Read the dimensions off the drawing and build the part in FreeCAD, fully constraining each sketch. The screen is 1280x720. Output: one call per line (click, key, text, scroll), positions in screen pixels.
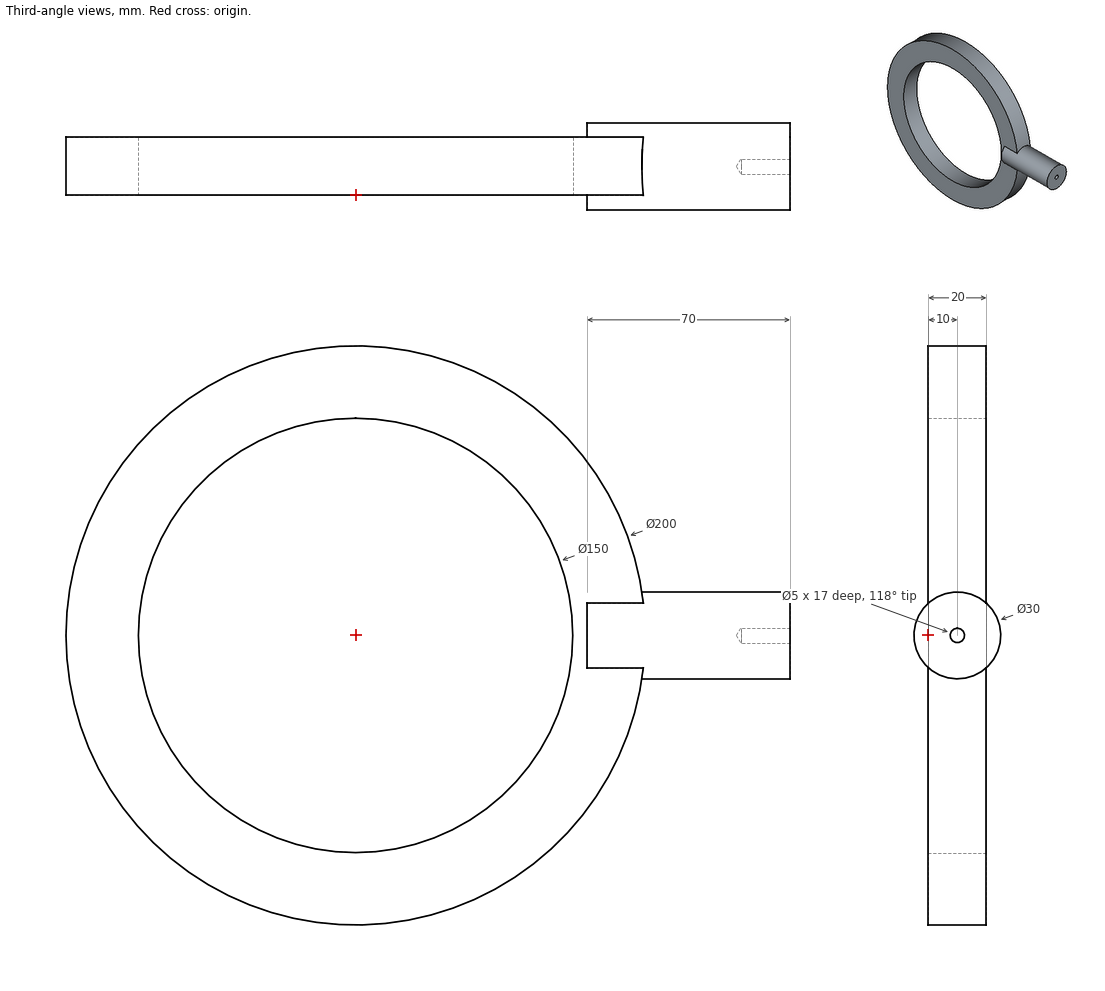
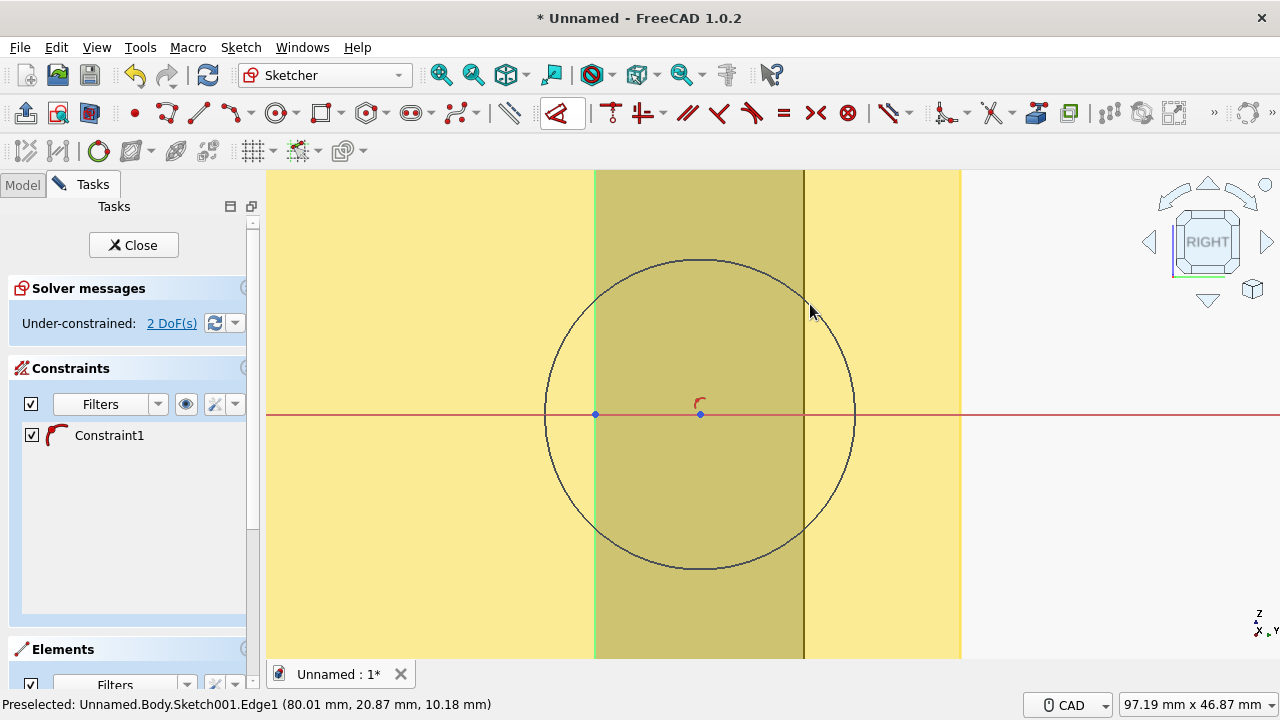
key(d)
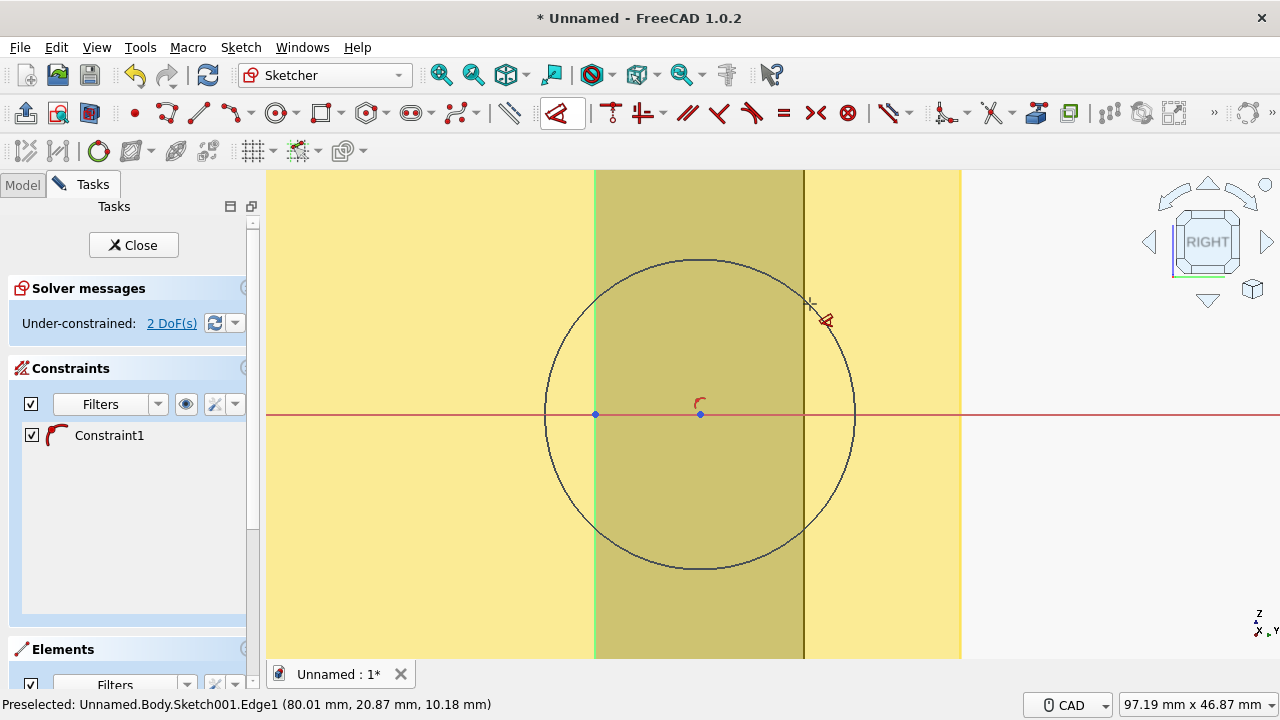
click(809, 304)
click(831, 281)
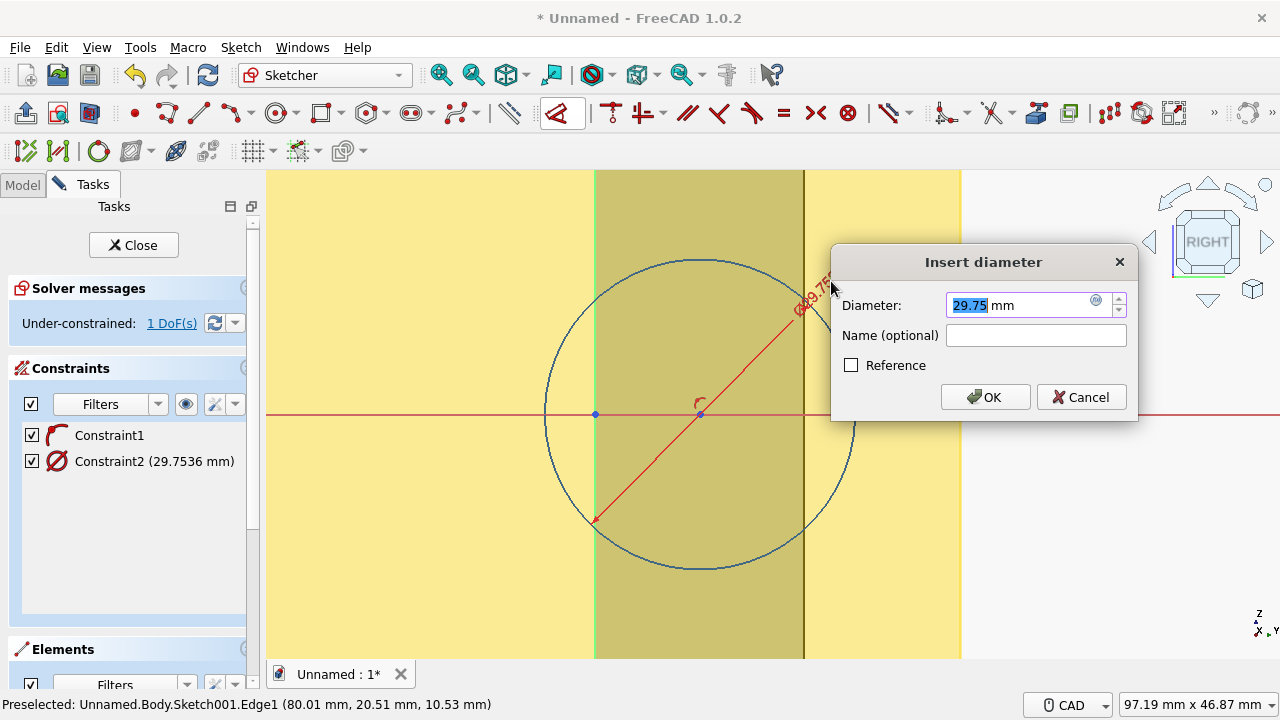
text(30)
key(Return)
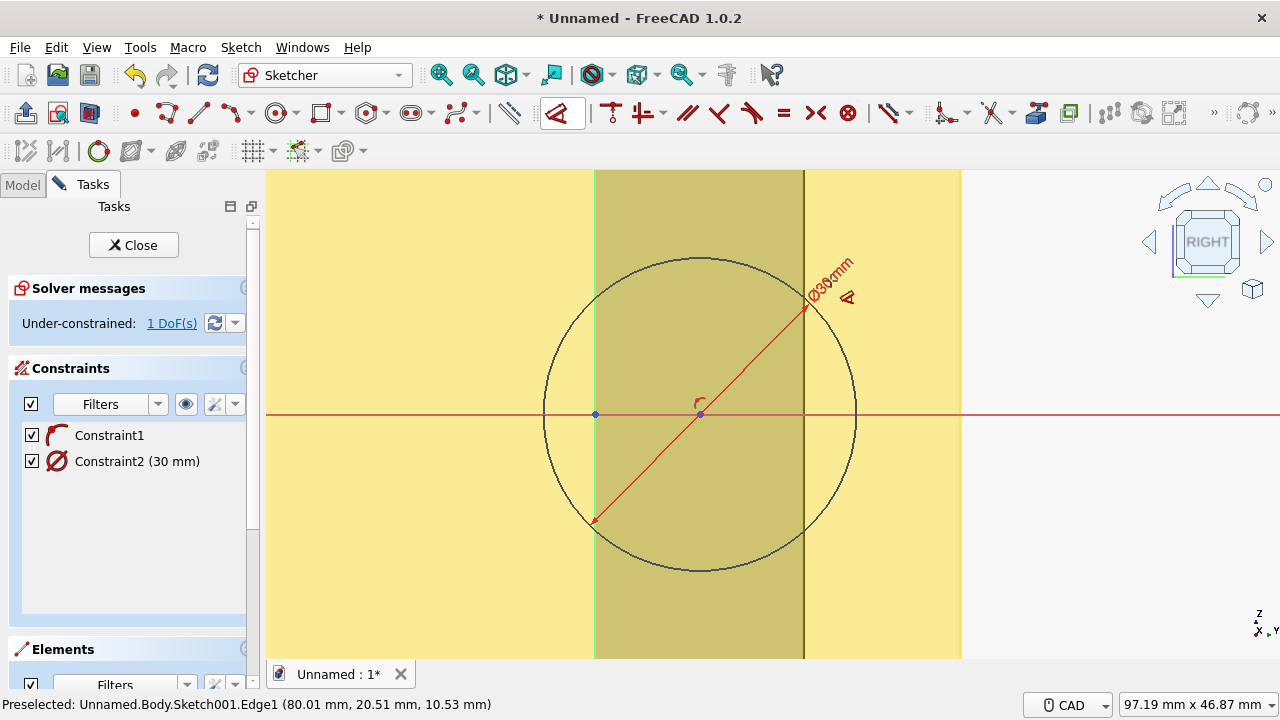
click(700, 414)
click(648, 448)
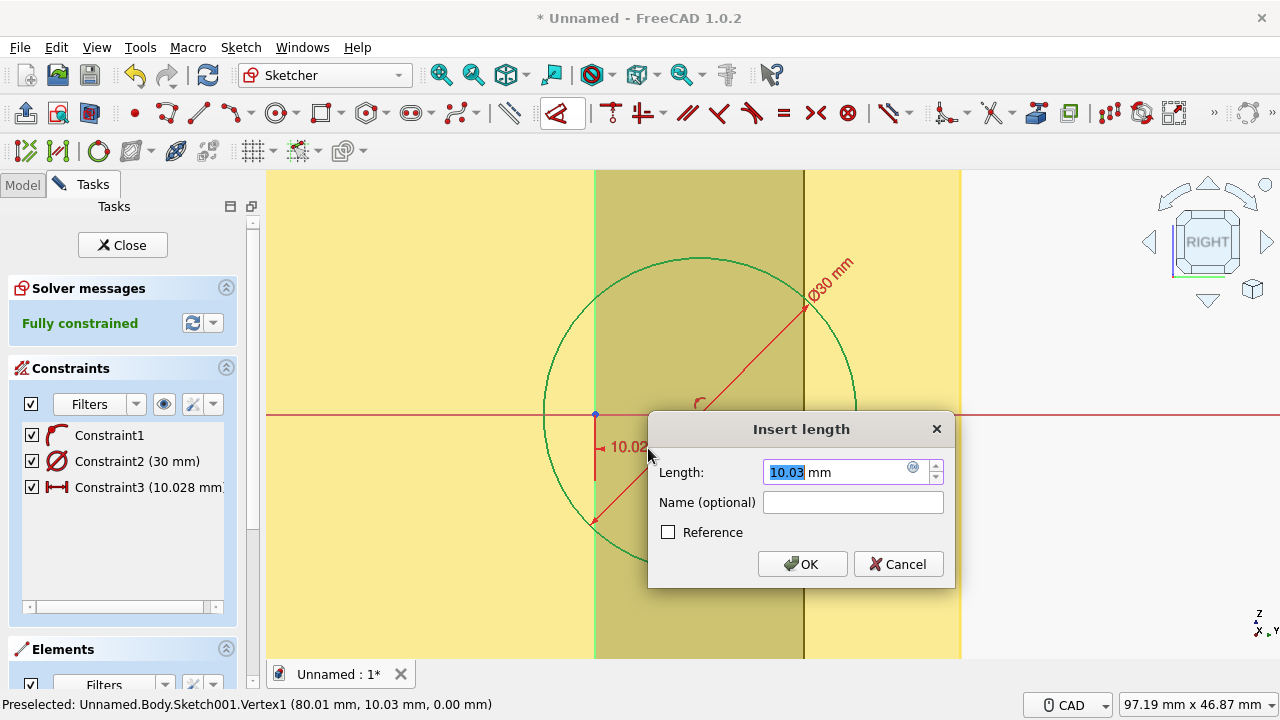
text(10)
key(Return)
key(Escape)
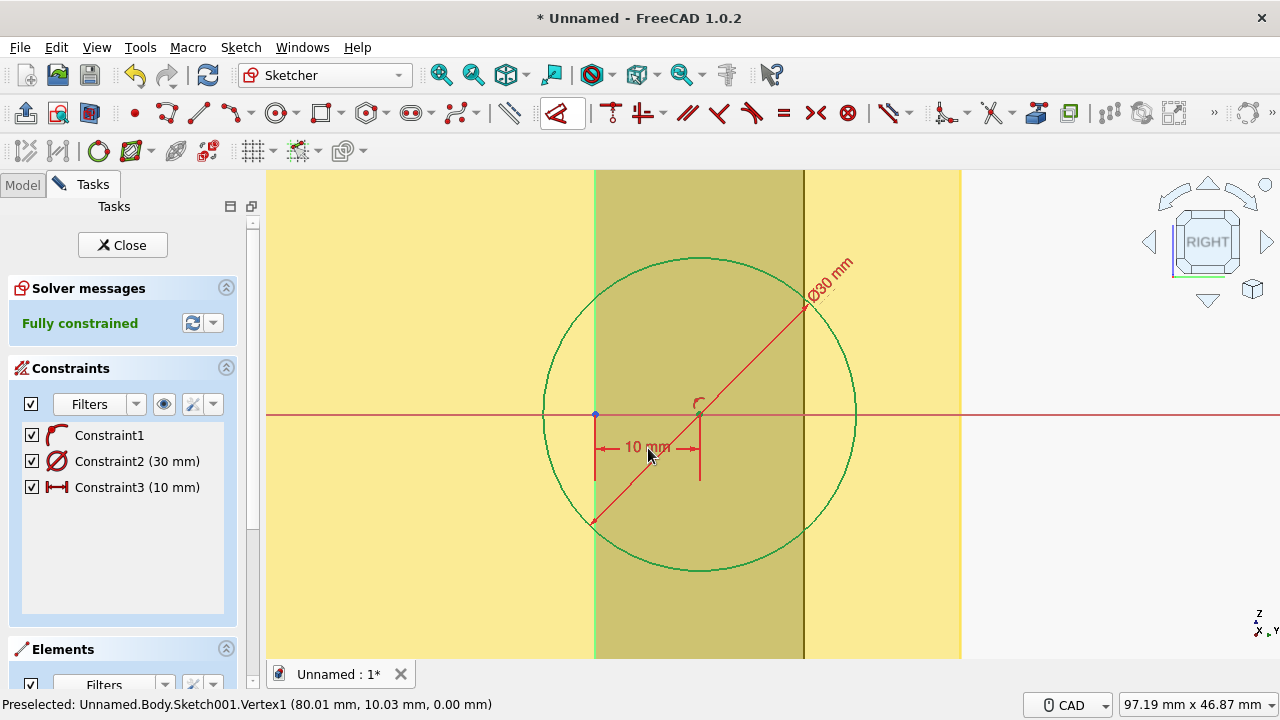
click(123, 245)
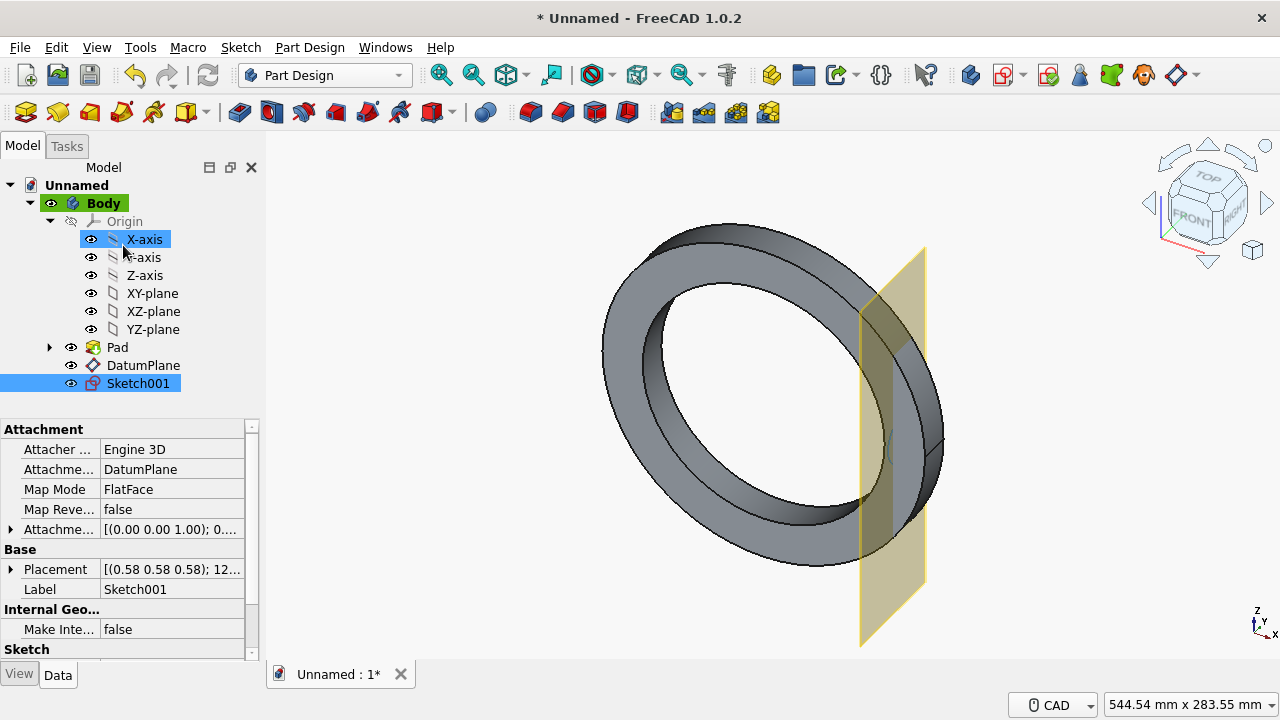
click(26, 112)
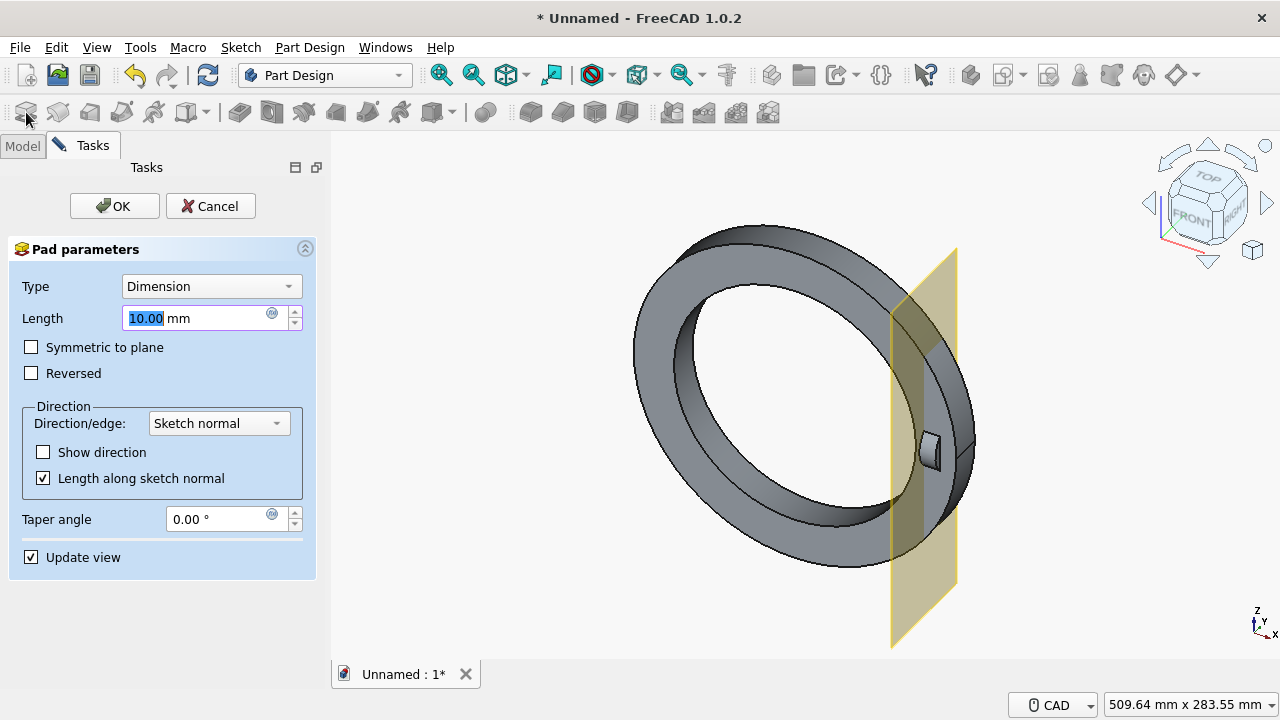
text(70)
key(Tab)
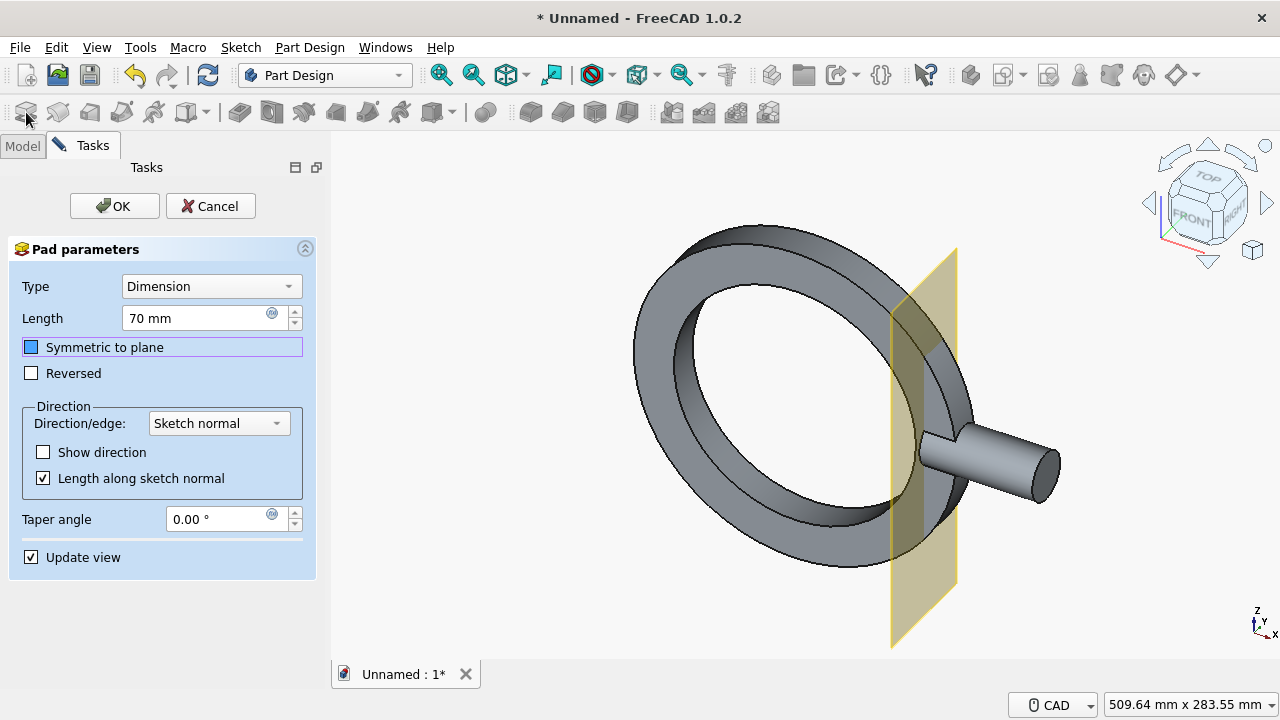
click(115, 206)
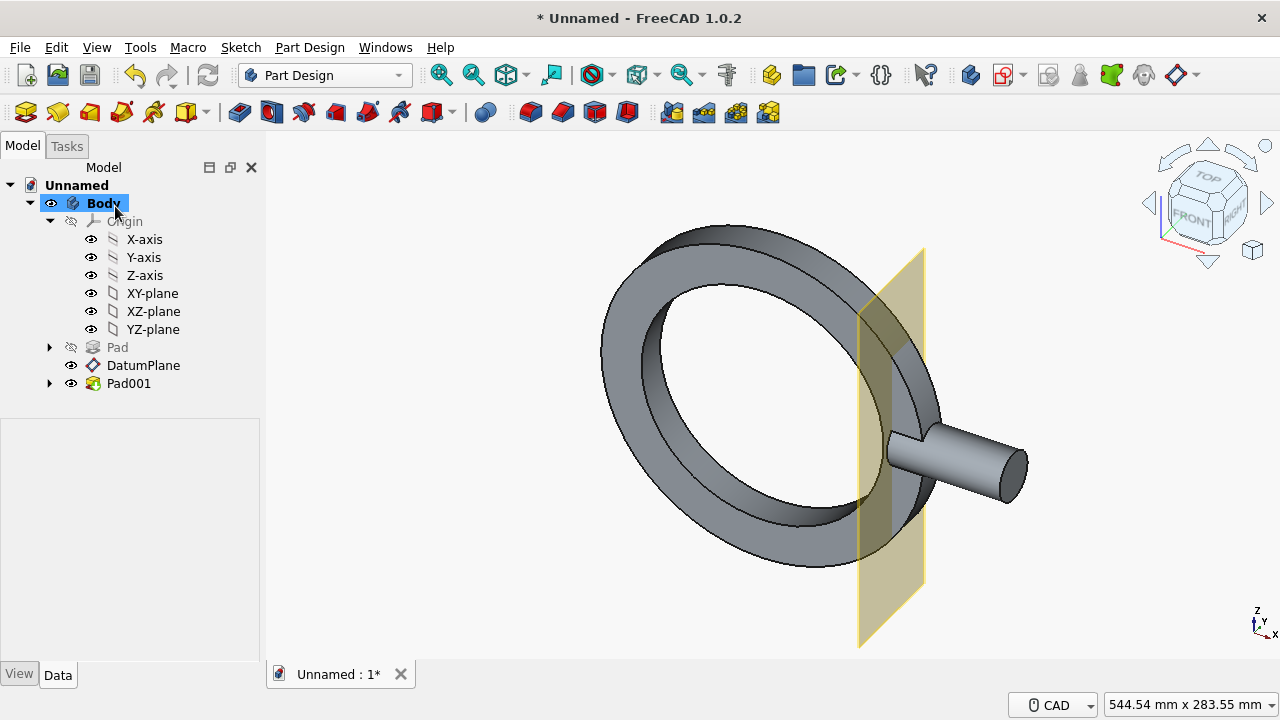
click(116, 365)
key(space)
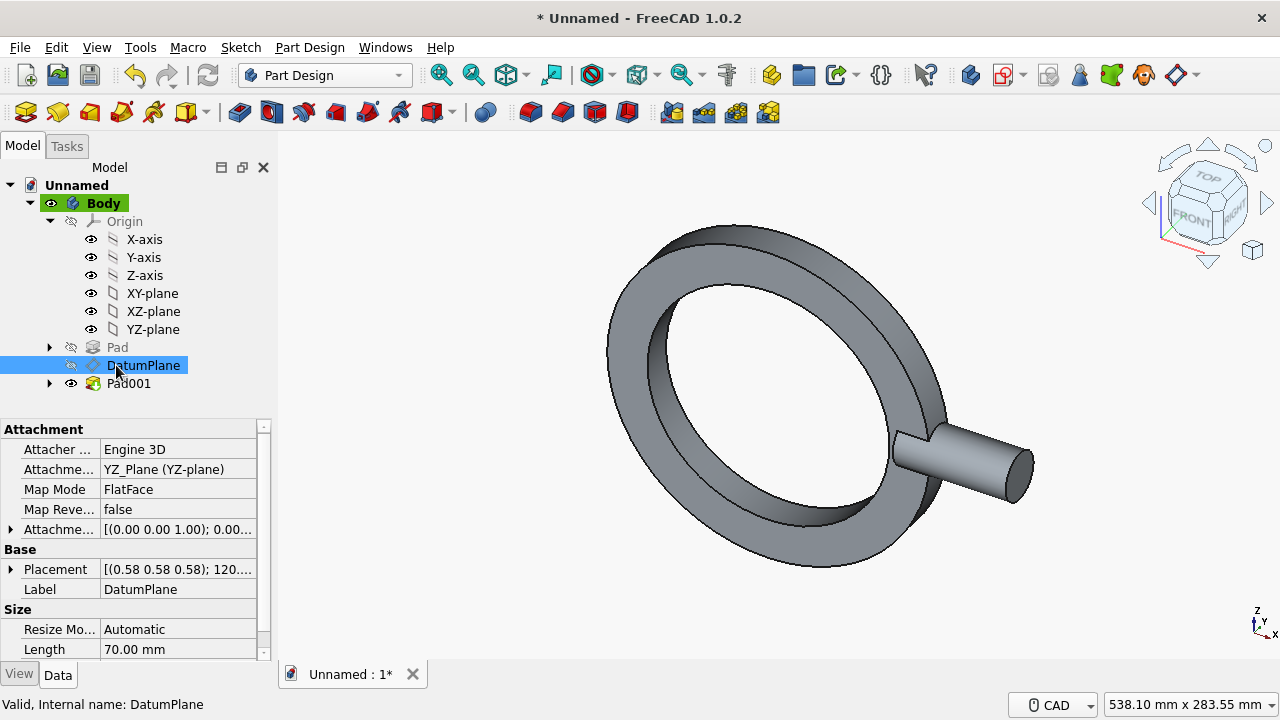
click(1020, 475)